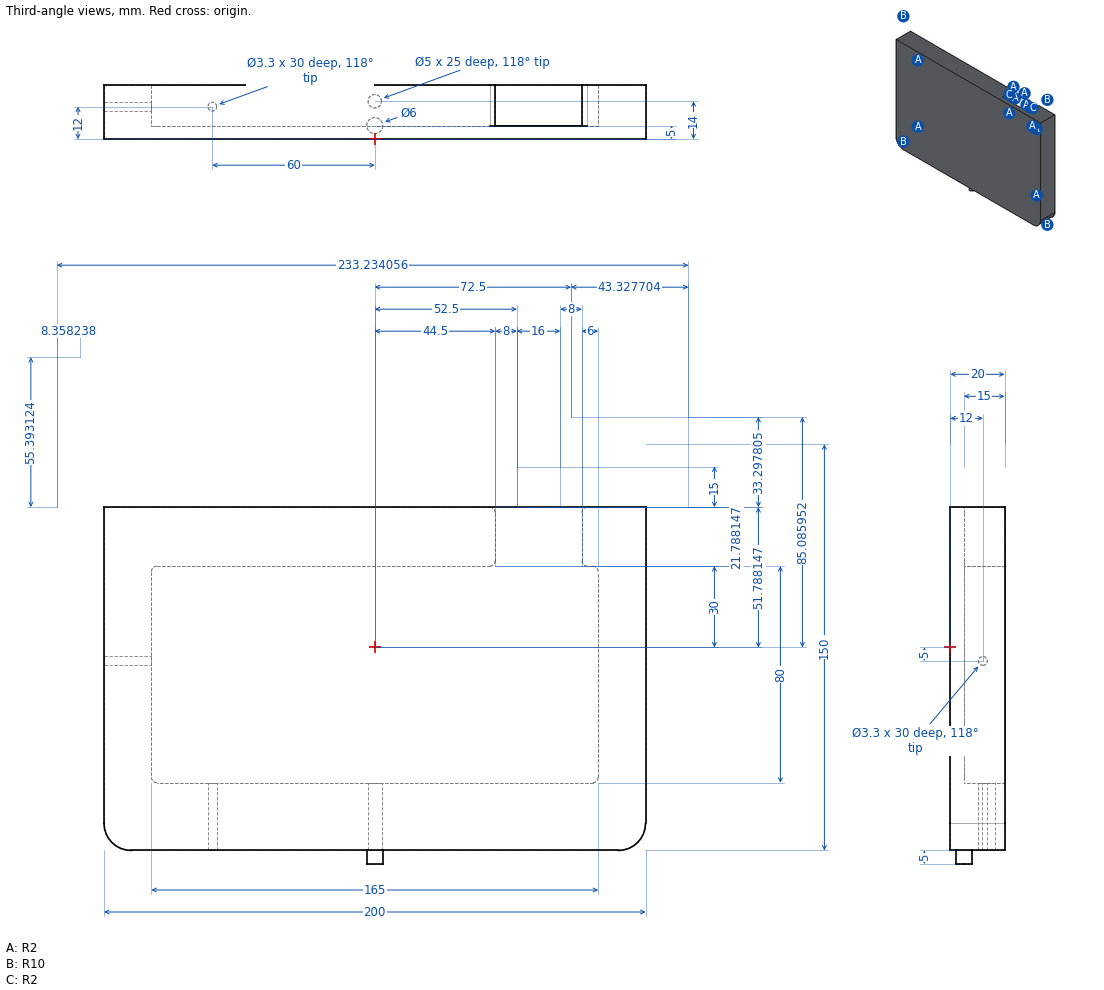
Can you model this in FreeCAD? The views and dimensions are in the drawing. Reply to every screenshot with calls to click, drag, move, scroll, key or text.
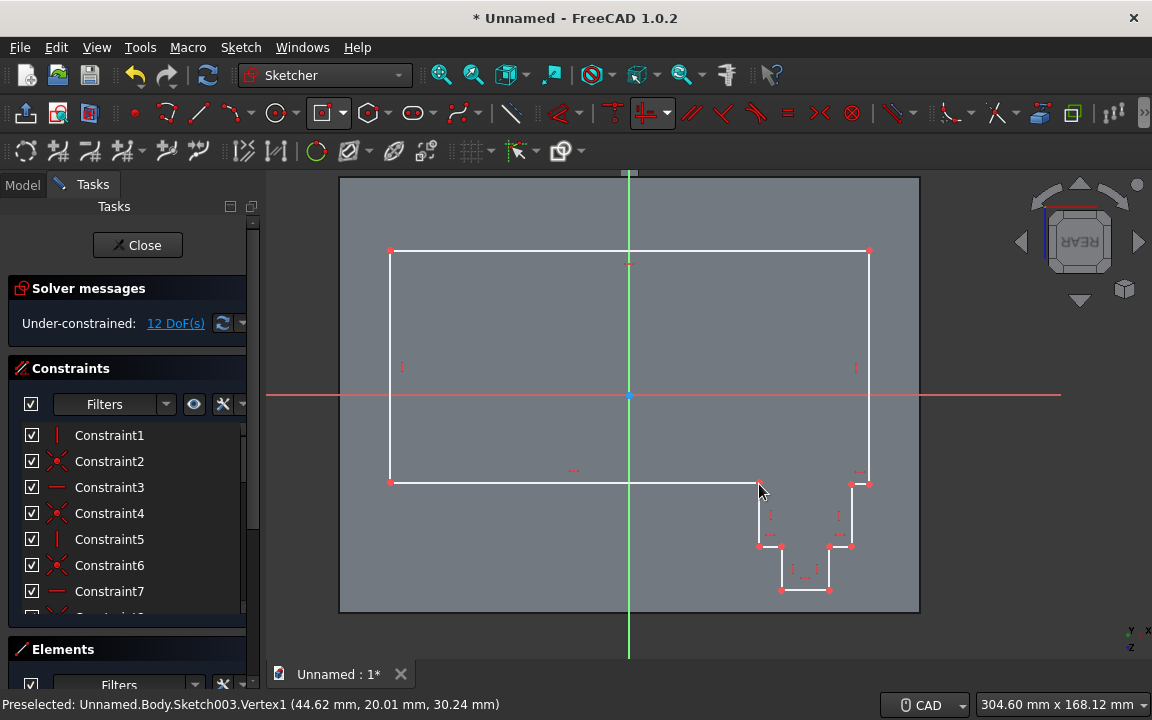
click(558, 114)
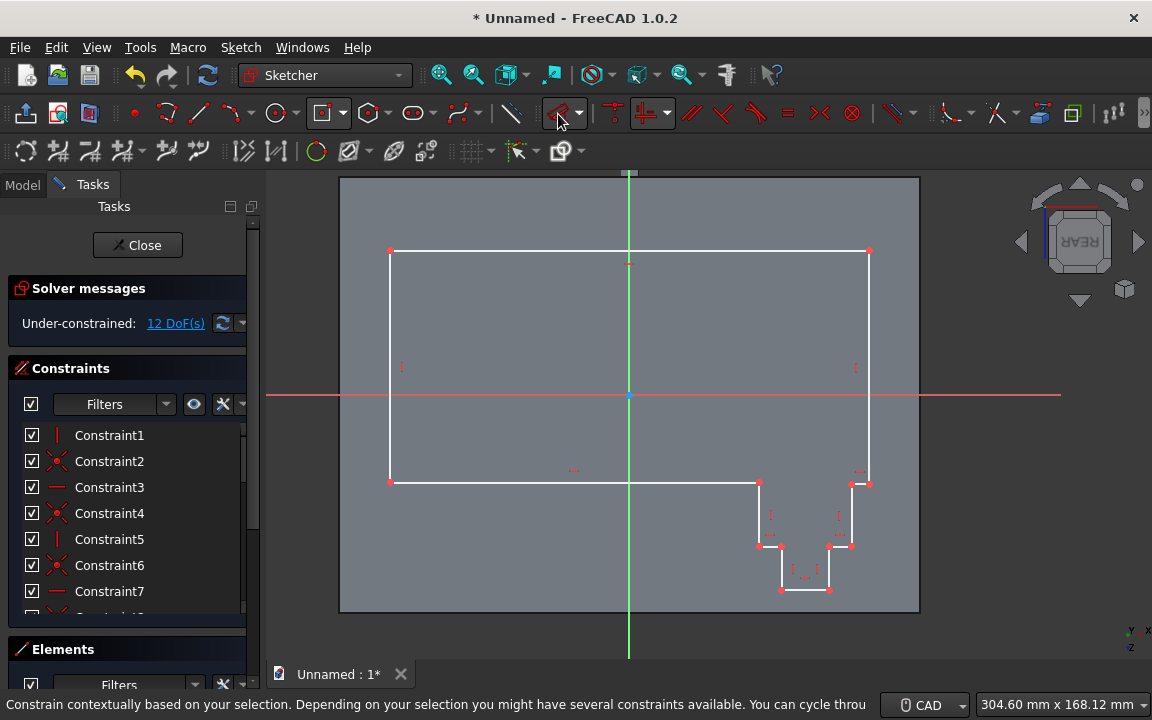
scroll(770, 547, up, 3)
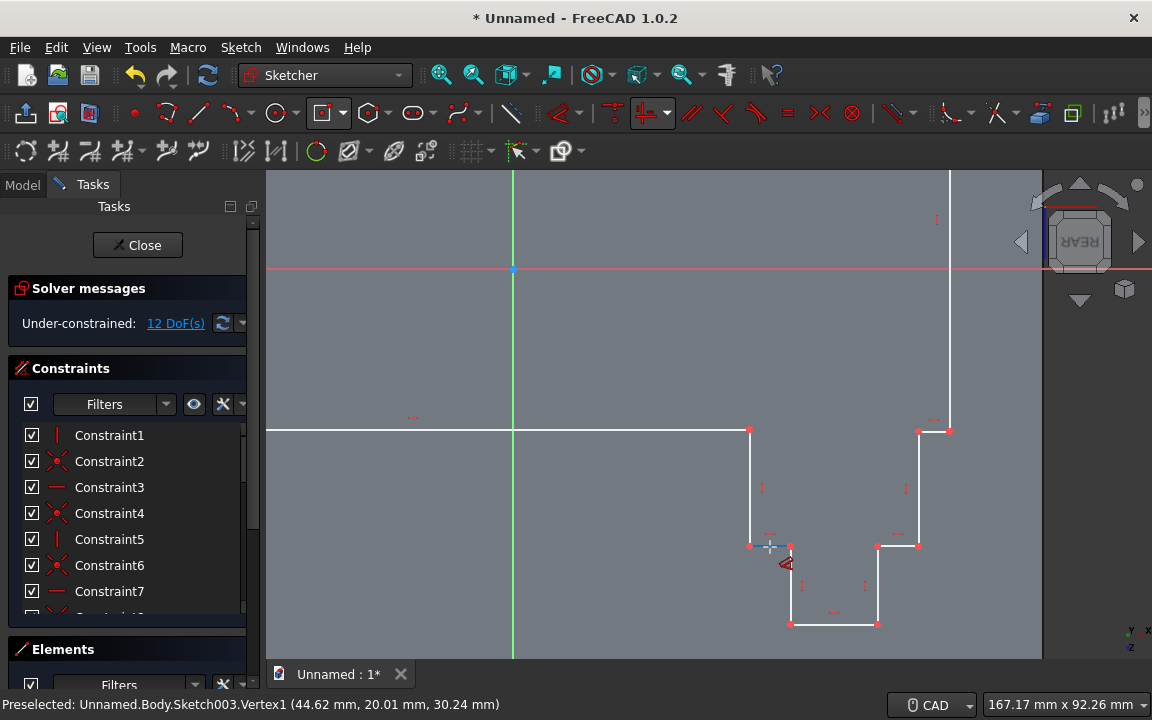
click(770, 546)
click(770, 580)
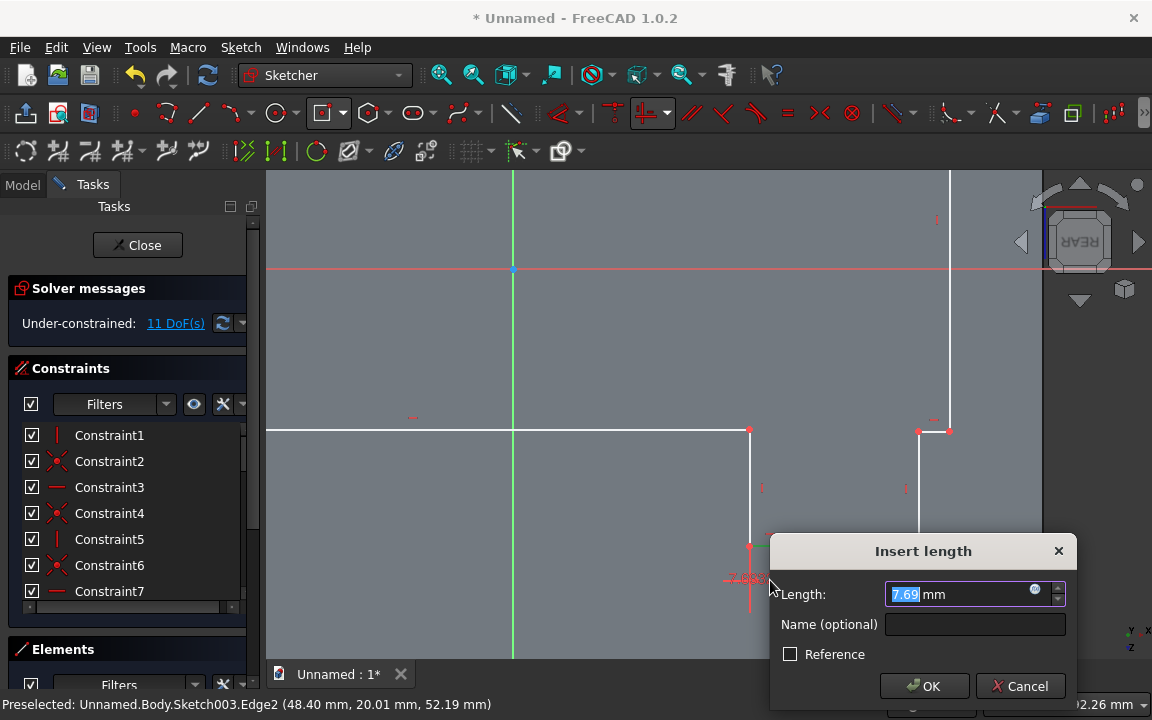
text(8)
key(Return)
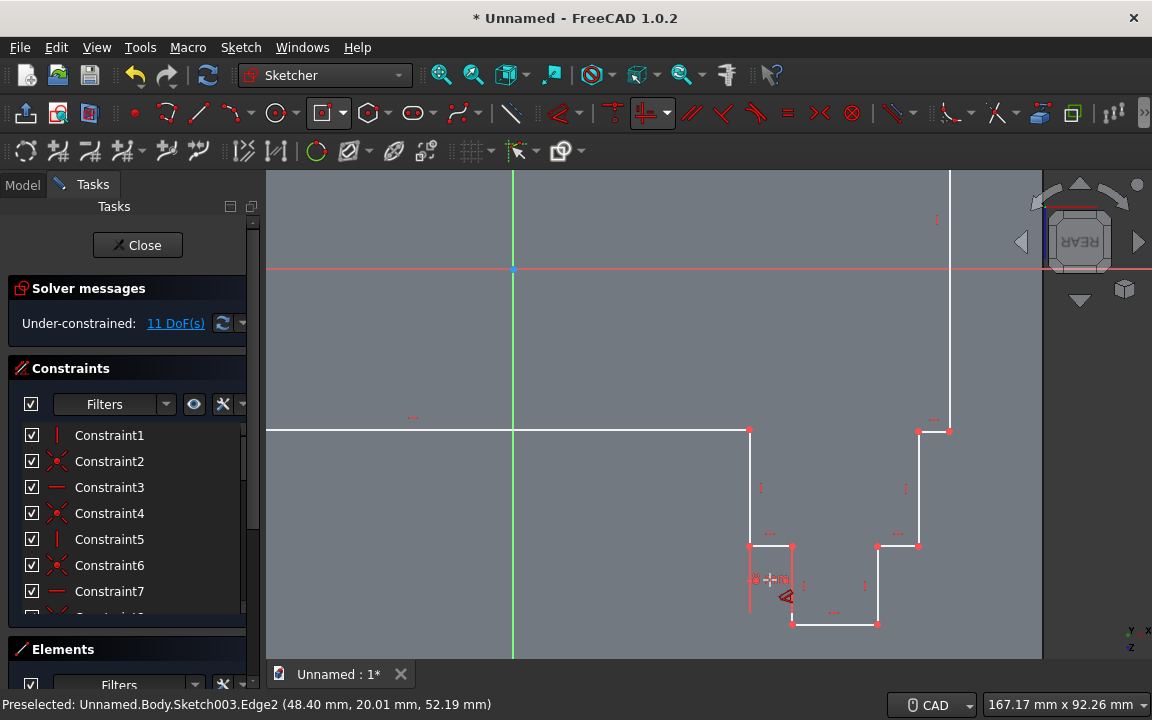
click(890, 546)
click(898, 580)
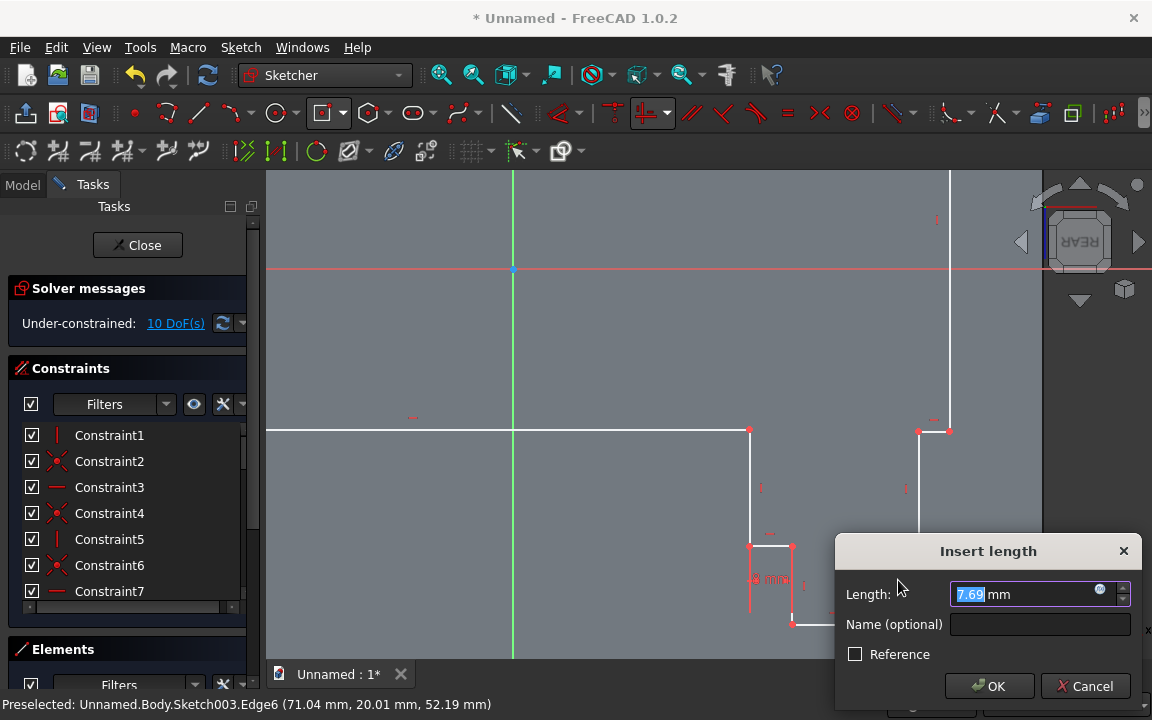
text(8)
key(Return)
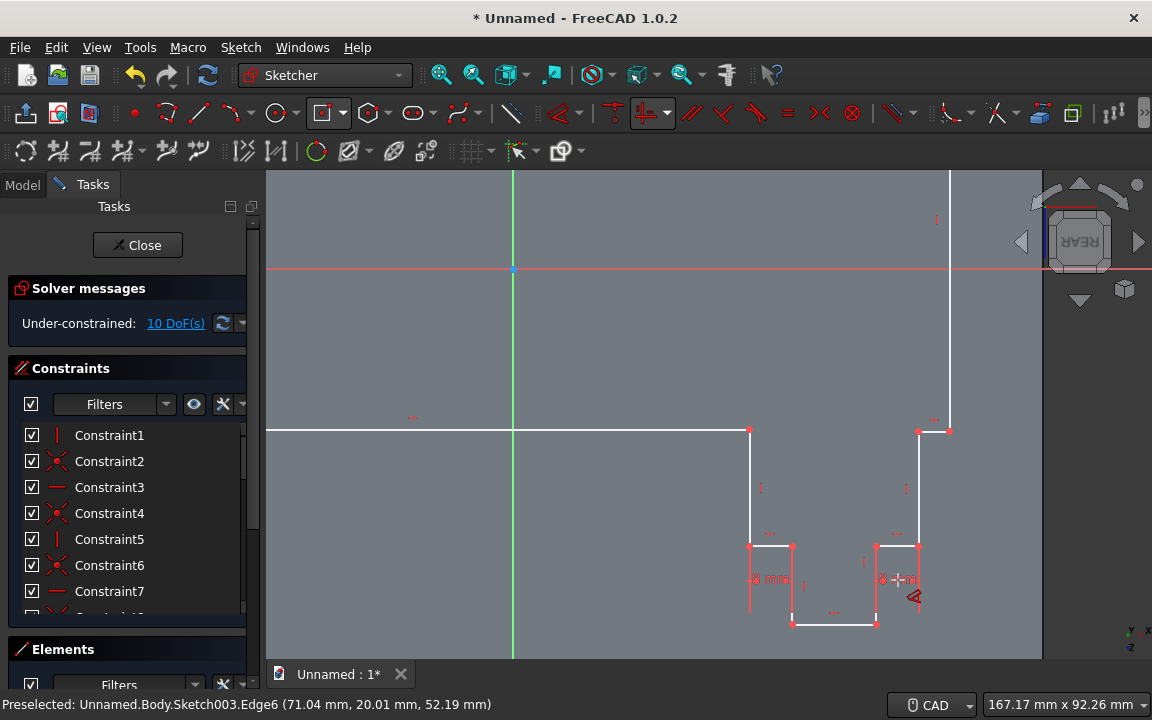
scroll(928, 432, up, 2)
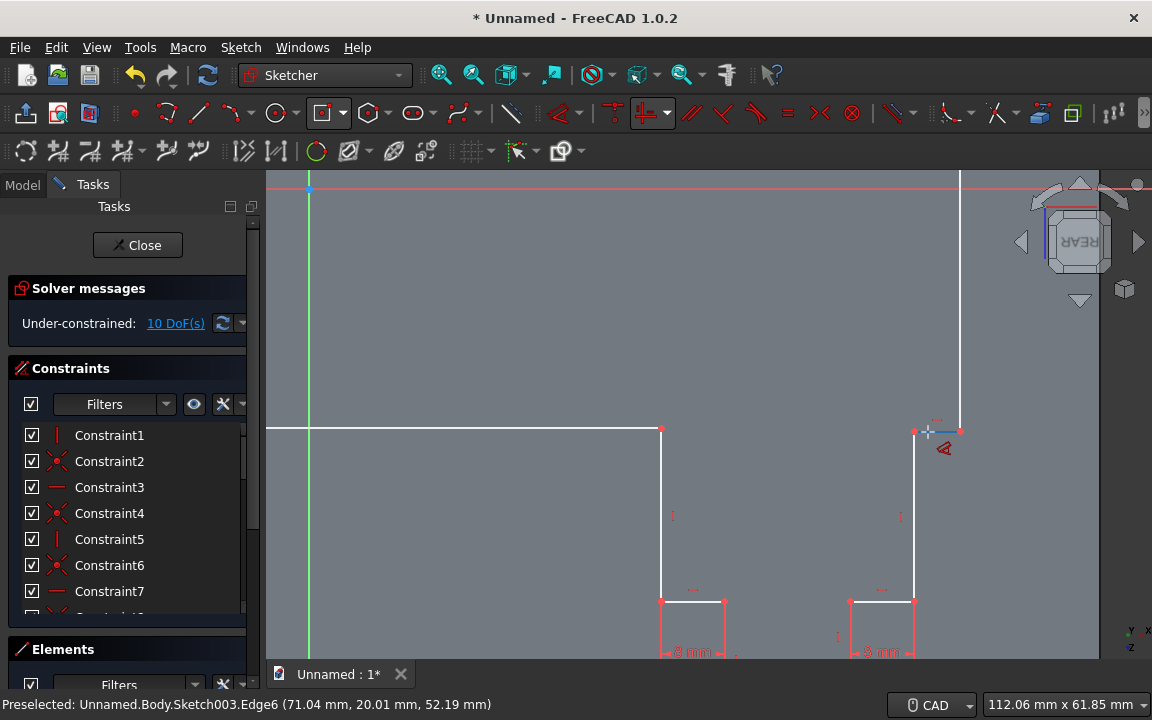
click(928, 432)
click(937, 466)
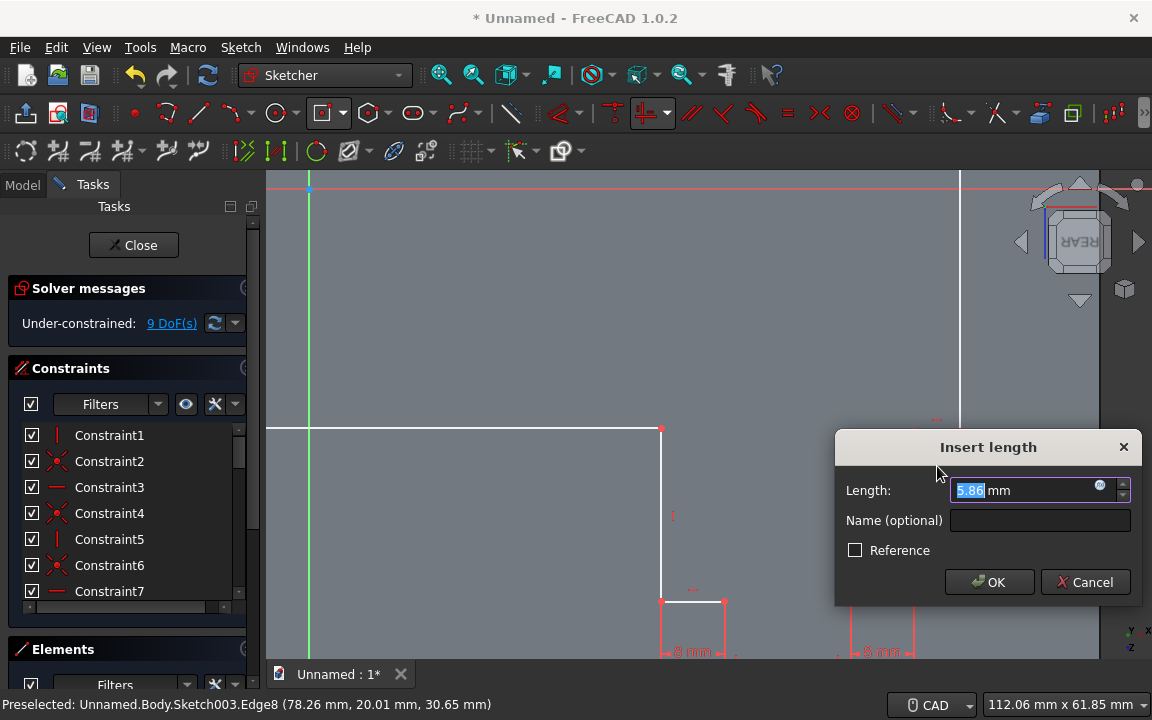
text(6)
key(Return)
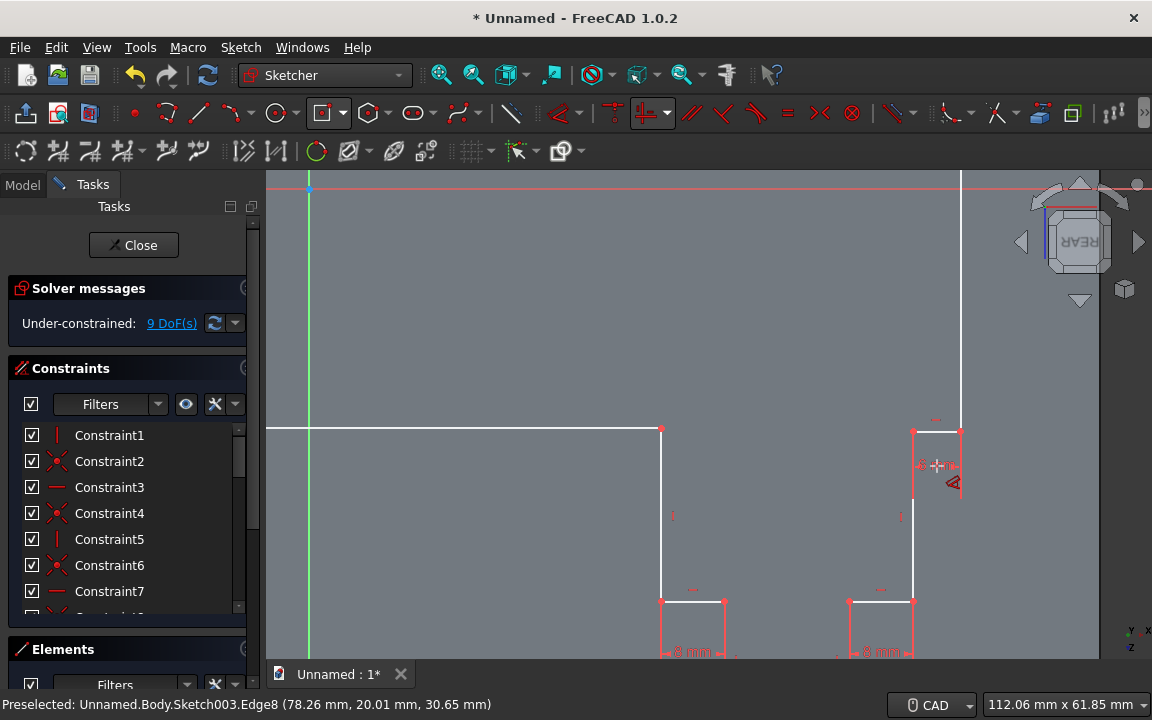
click(725, 625)
click(759, 616)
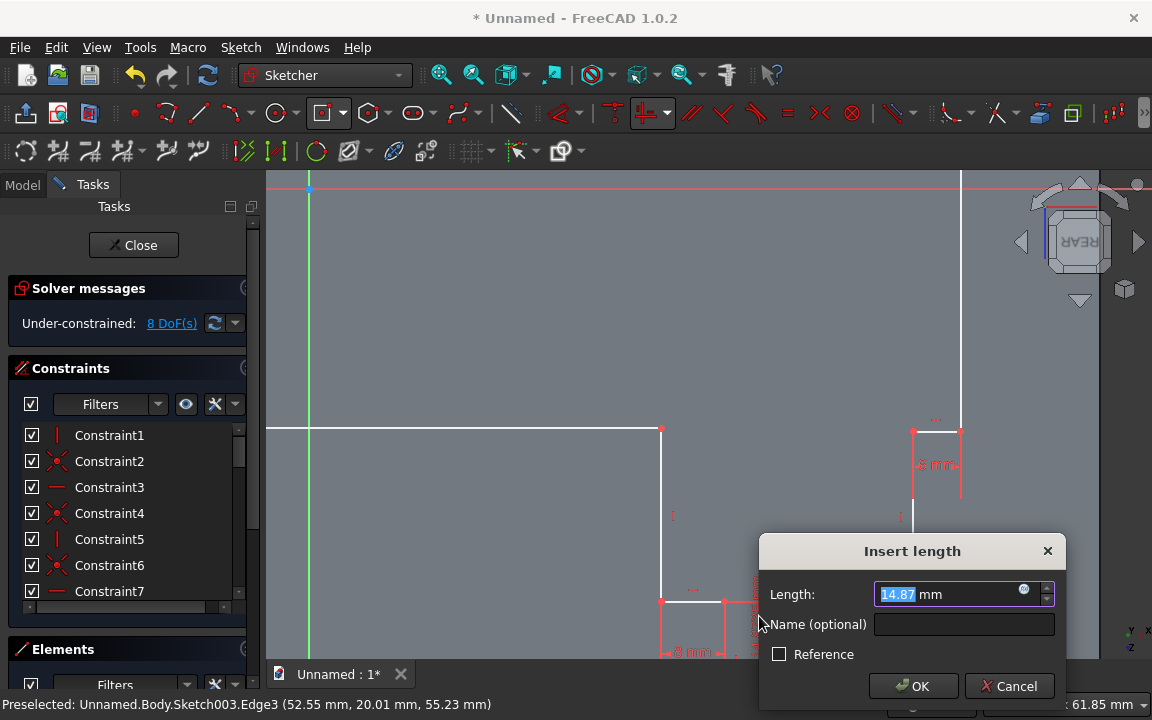
text(15)
key(Return)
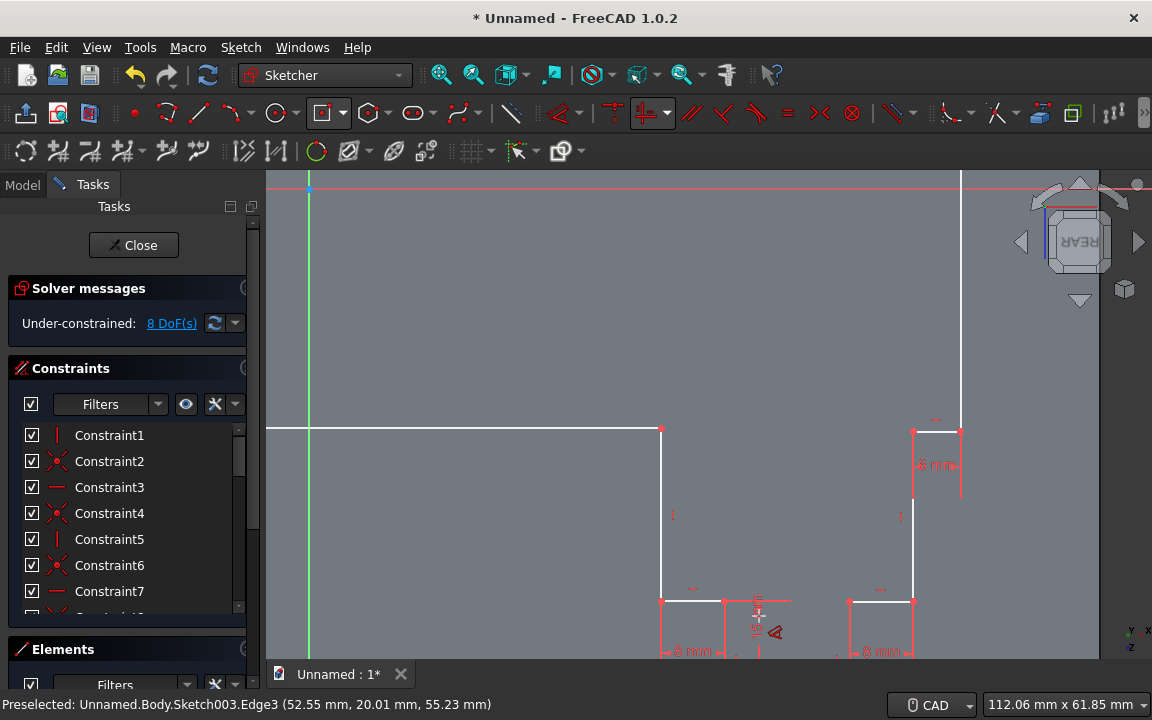
scroll(783, 483, down, 6)